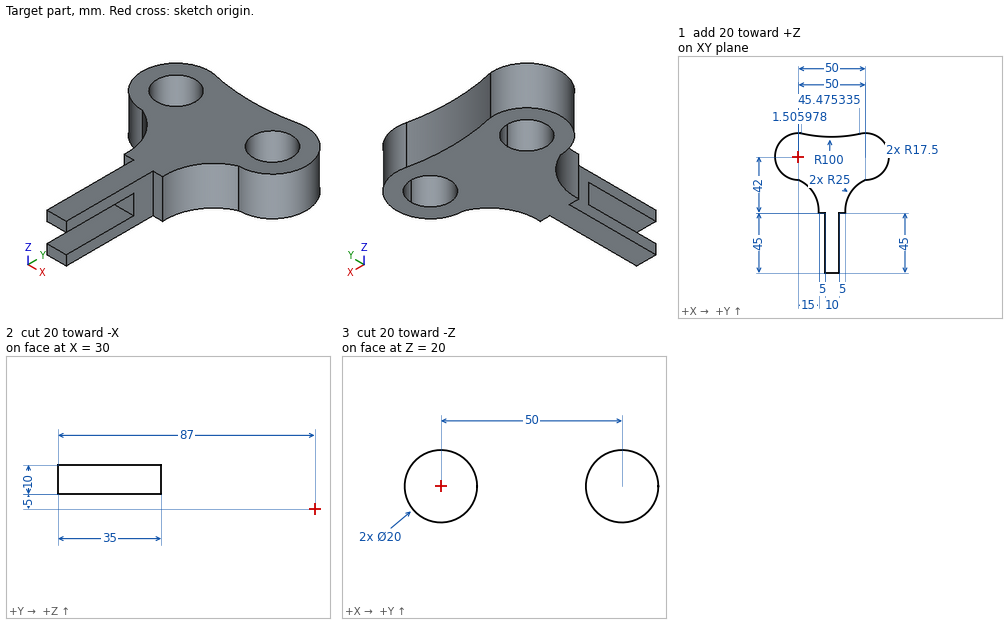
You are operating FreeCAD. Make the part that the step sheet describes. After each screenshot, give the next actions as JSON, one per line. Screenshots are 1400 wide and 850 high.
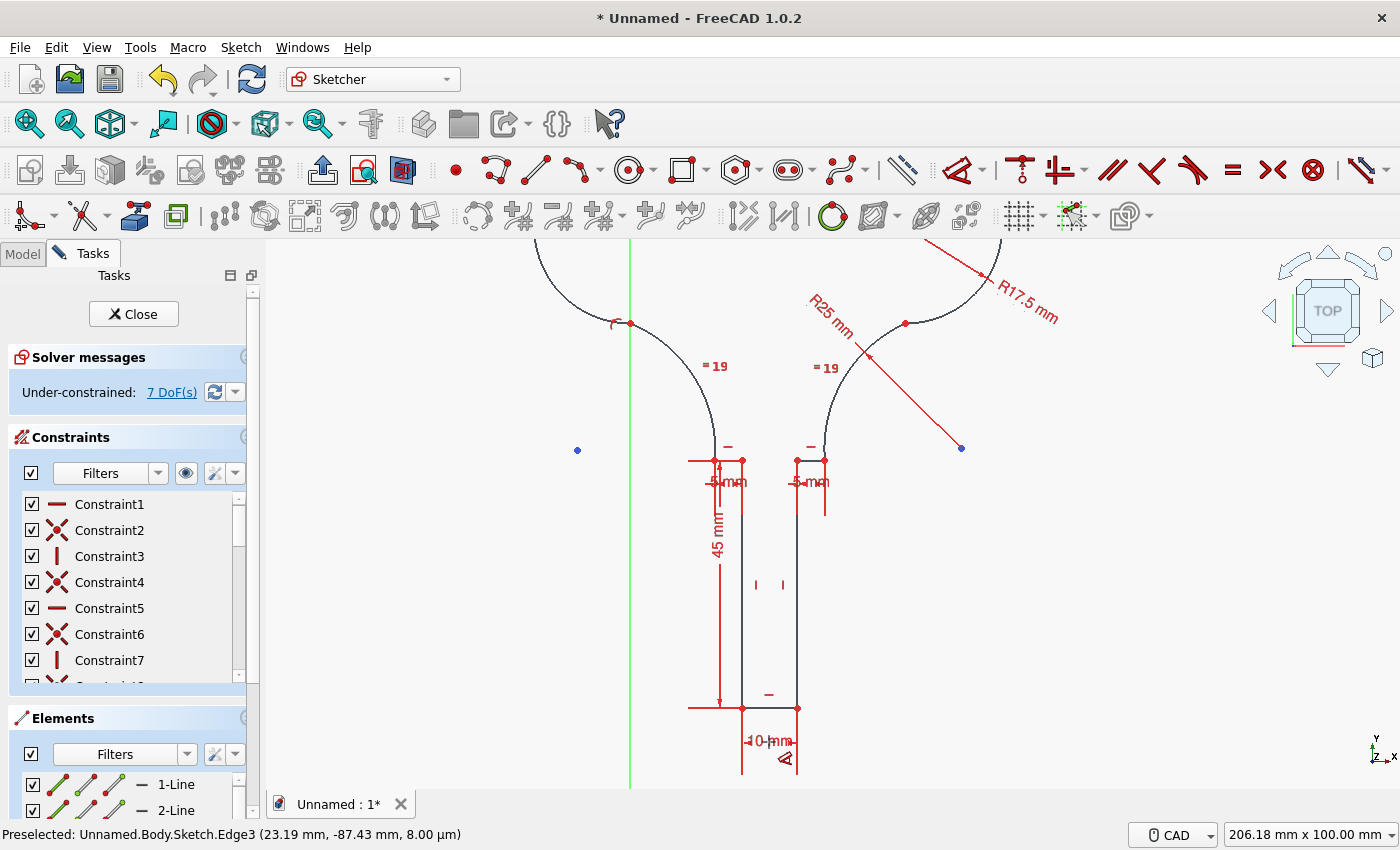
{"action": "left_click", "coordinate": [797, 634]}
{"action": "left_click", "coordinate": [831, 584]}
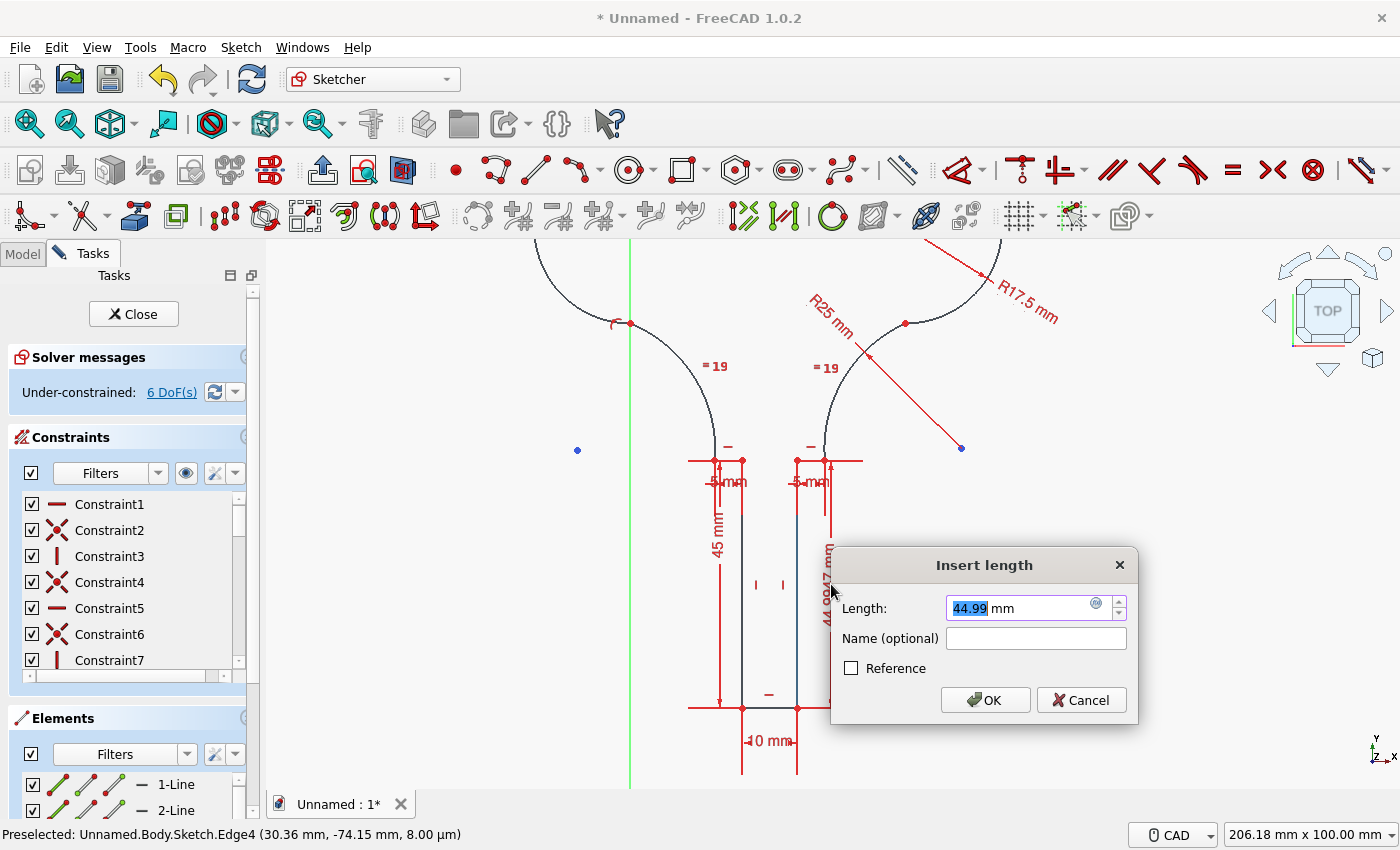
{"action": "type", "text": "45"}
{"action": "key", "text": "Return"}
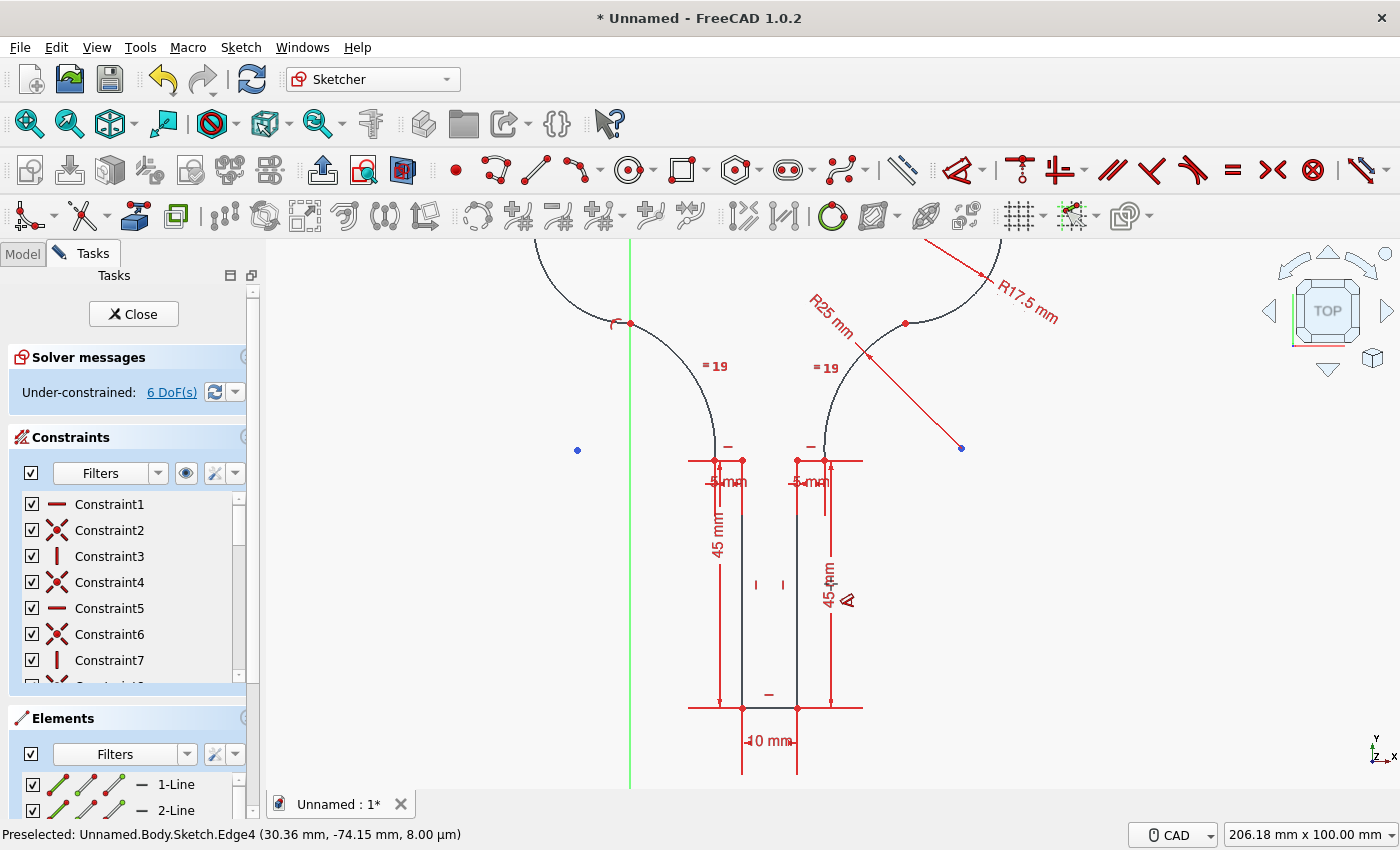
{"action": "left_click", "coordinate": [715, 461]}
{"action": "left_click", "coordinate": [653, 495]}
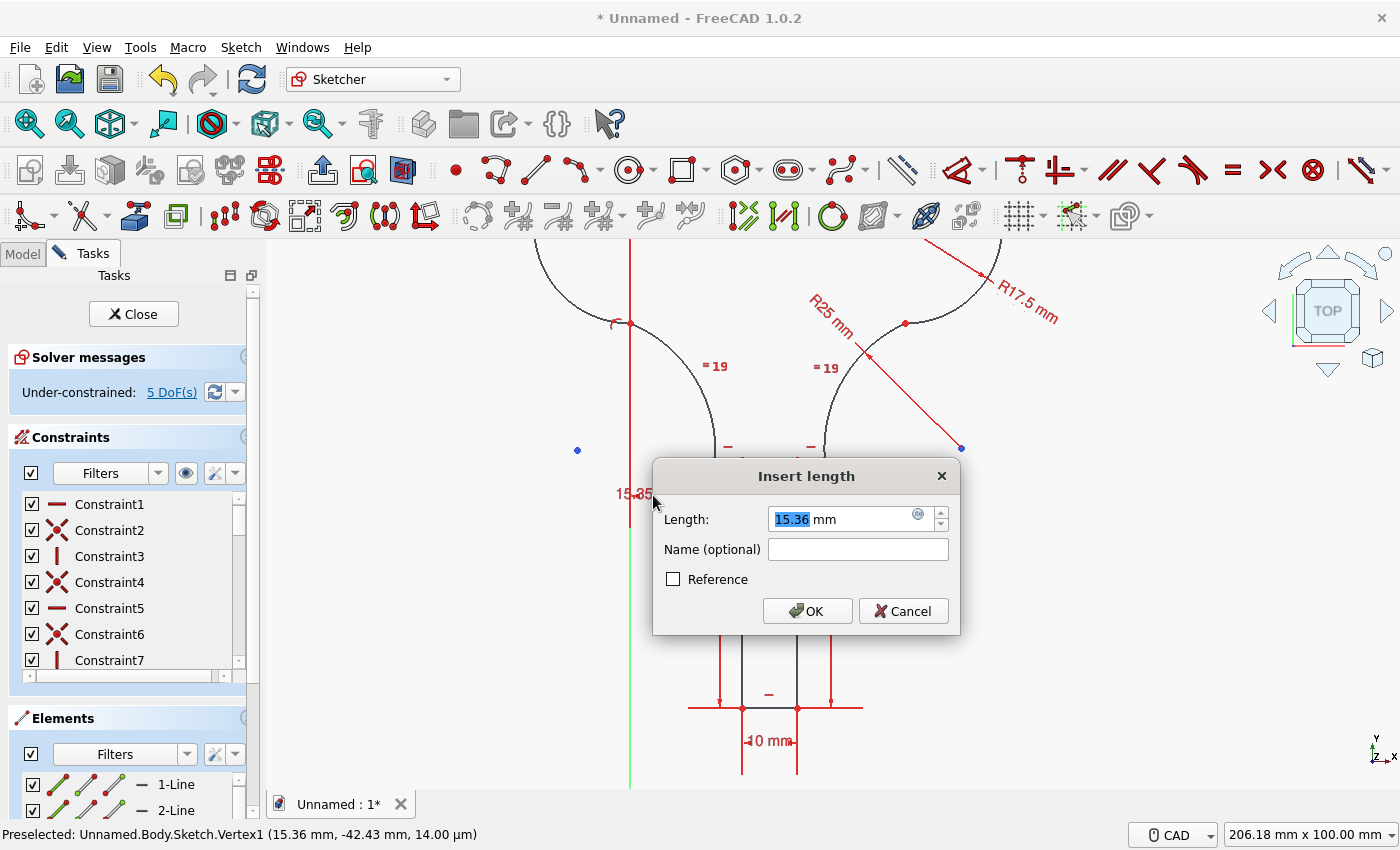
{"action": "type", "text": "15"}
{"action": "key", "text": "Return"}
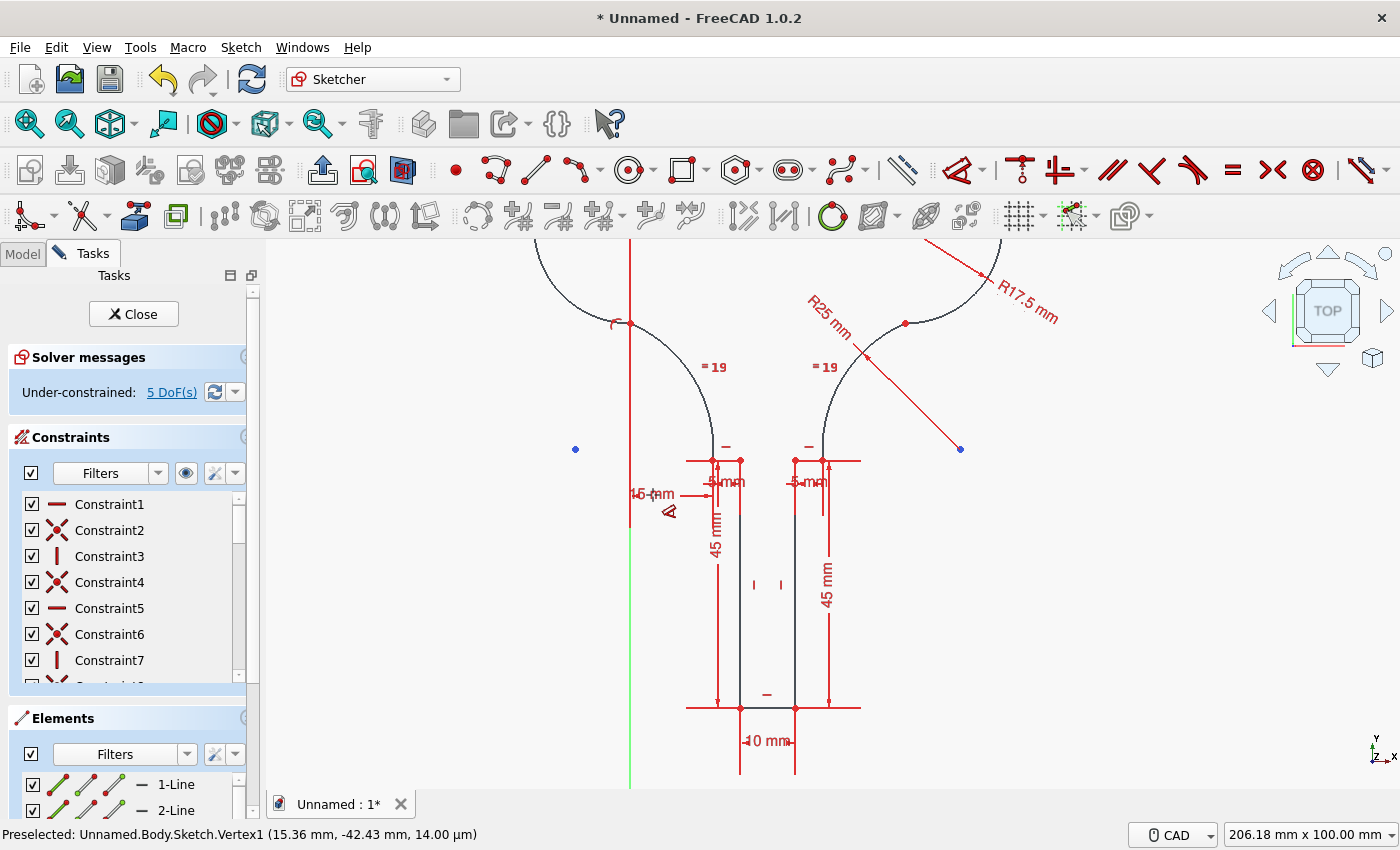
{"action": "left_click", "coordinate": [713, 461]}
{"action": "left_click", "coordinate": [596, 364]}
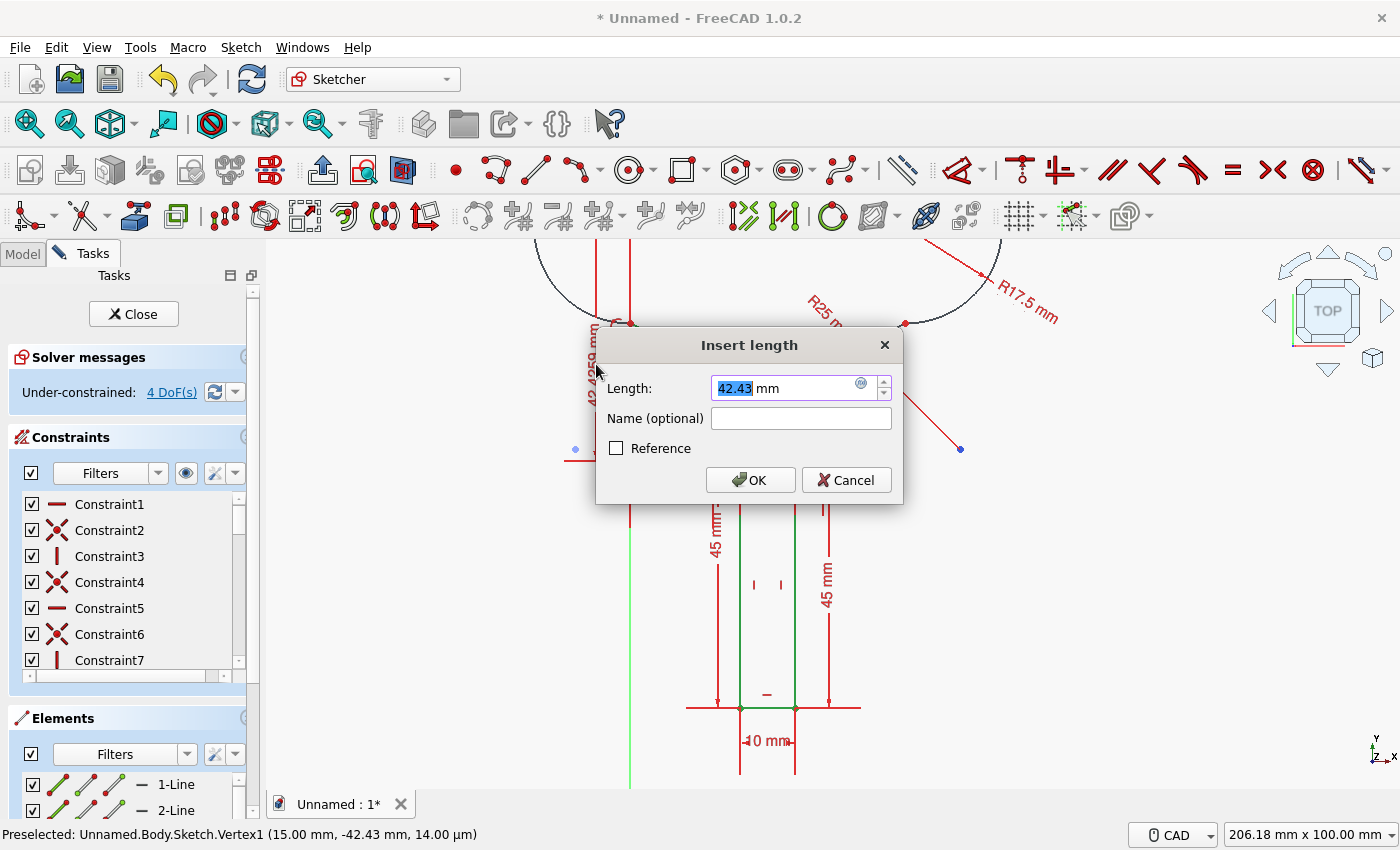
{"action": "type", "text": "42"}
{"action": "key", "text": "Return"}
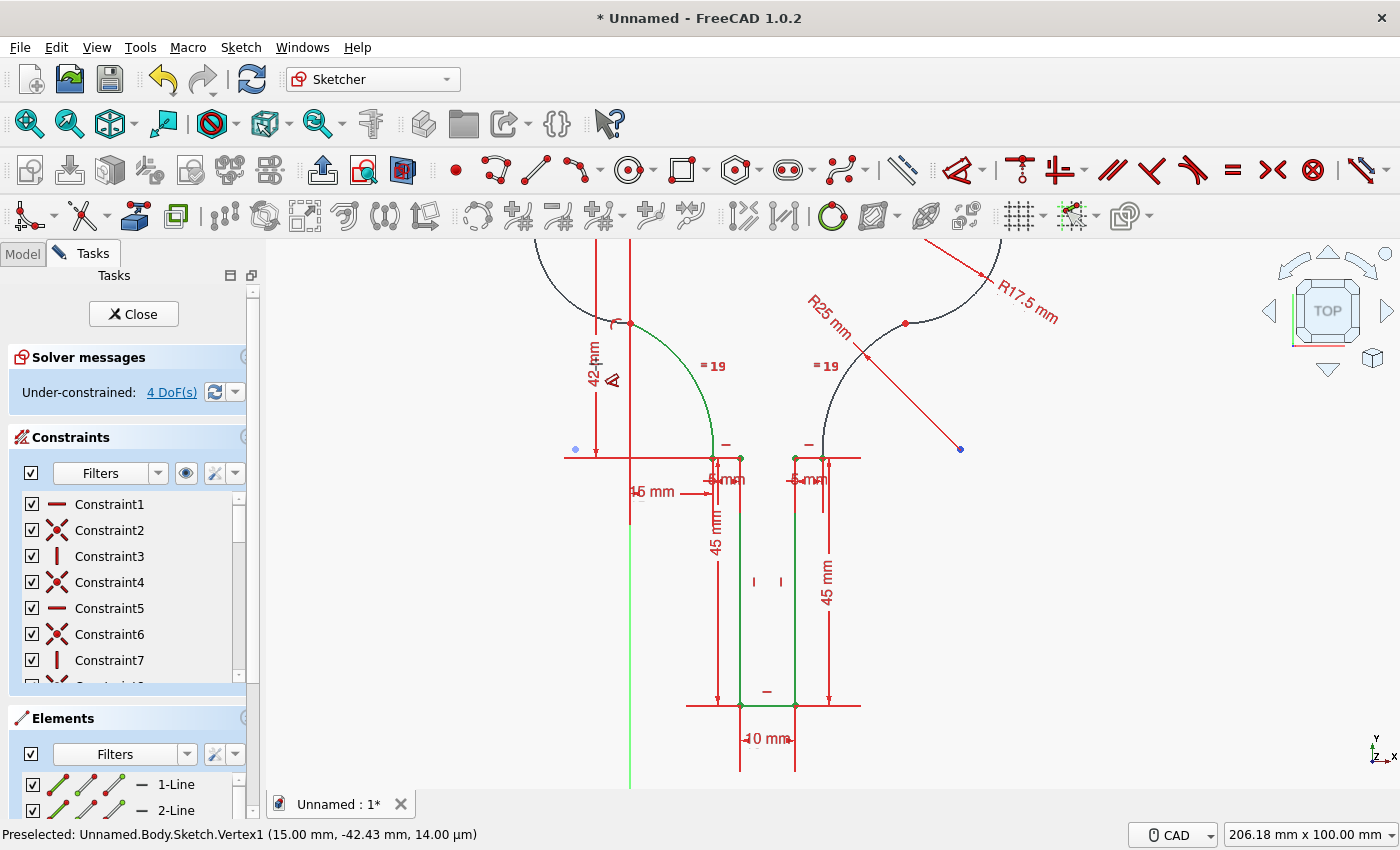
{"action": "left_click", "coordinate": [905, 323]}
{"action": "left_click", "coordinate": [768, 357]}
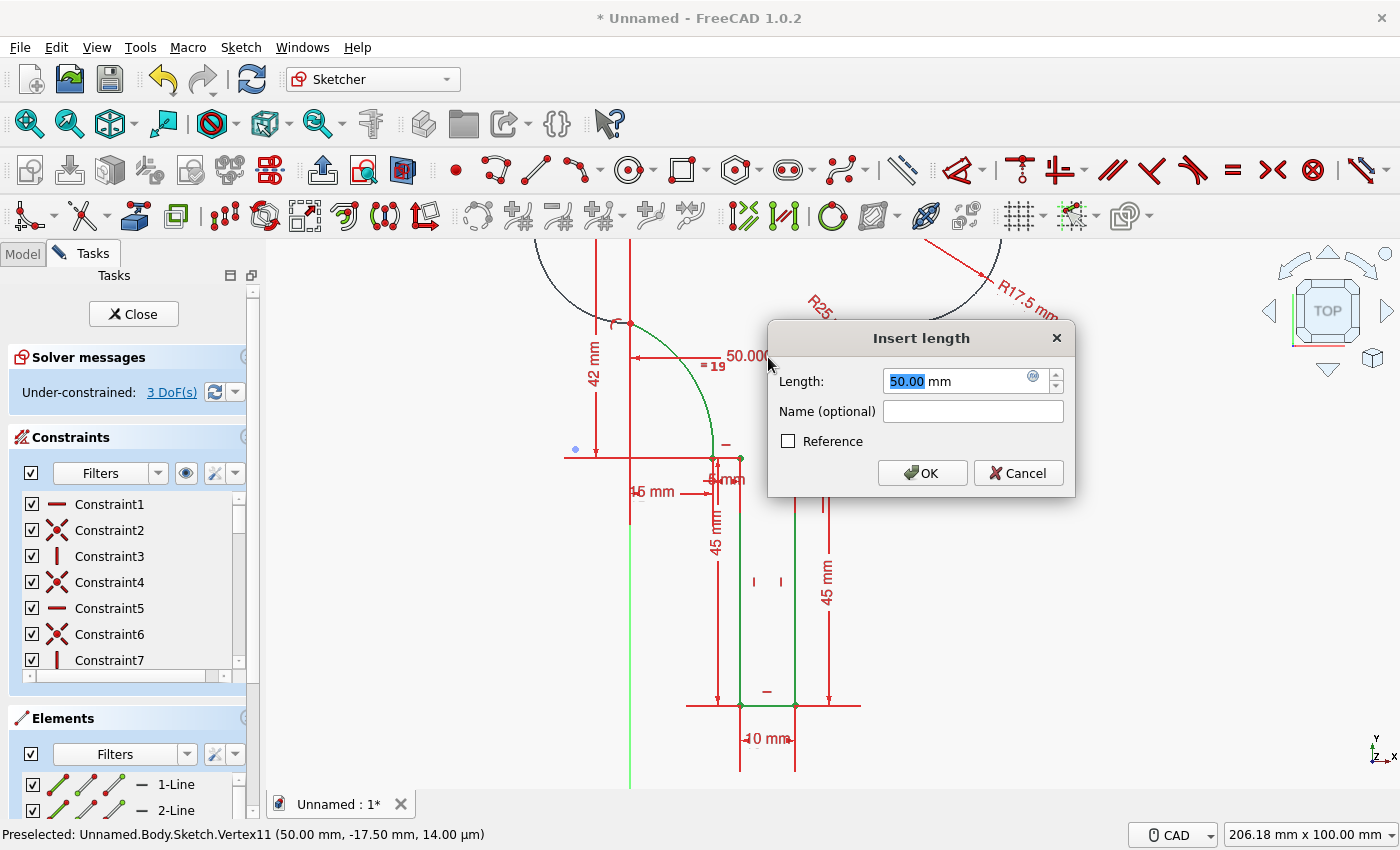
{"action": "type", "text": "50"}
{"action": "key", "text": "Return"}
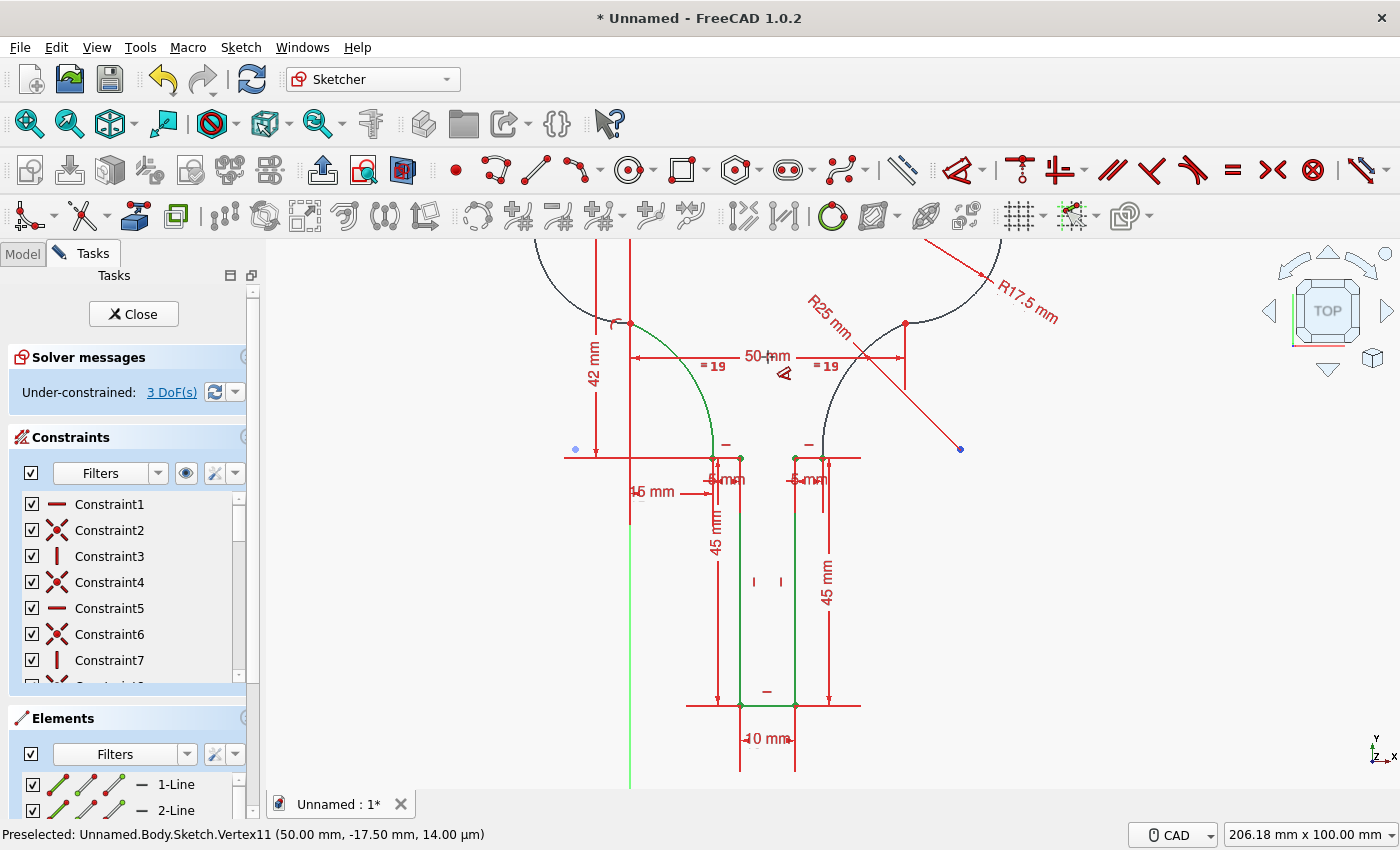
{"action": "scroll", "coordinate": [758, 708], "scroll_direction": "down", "scroll_amount": 2}